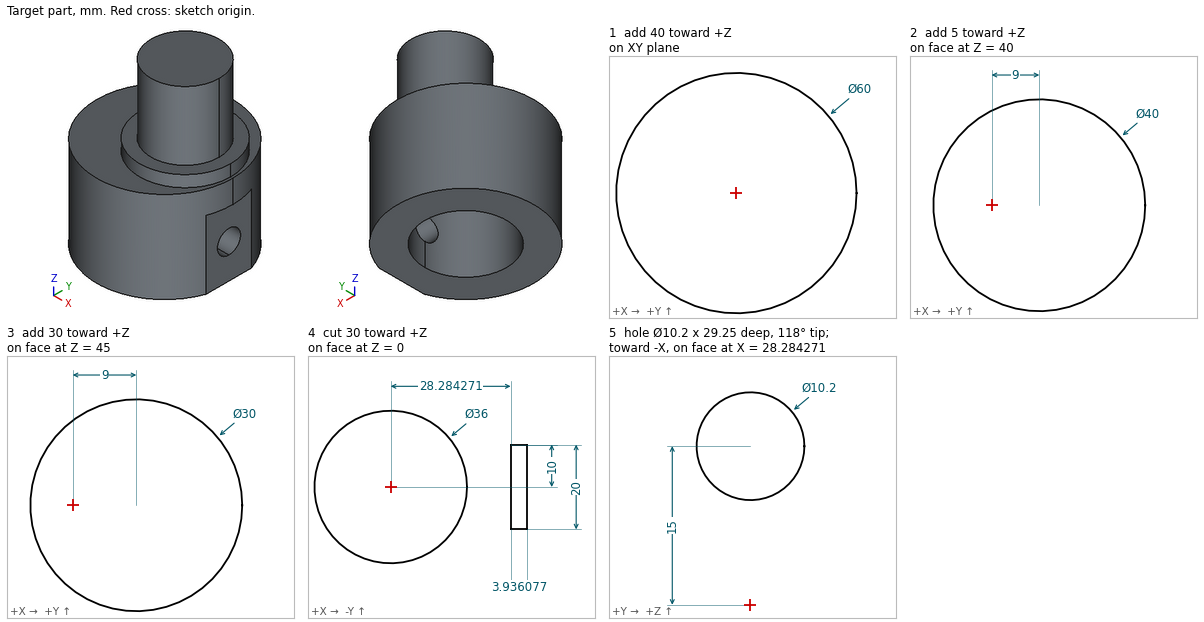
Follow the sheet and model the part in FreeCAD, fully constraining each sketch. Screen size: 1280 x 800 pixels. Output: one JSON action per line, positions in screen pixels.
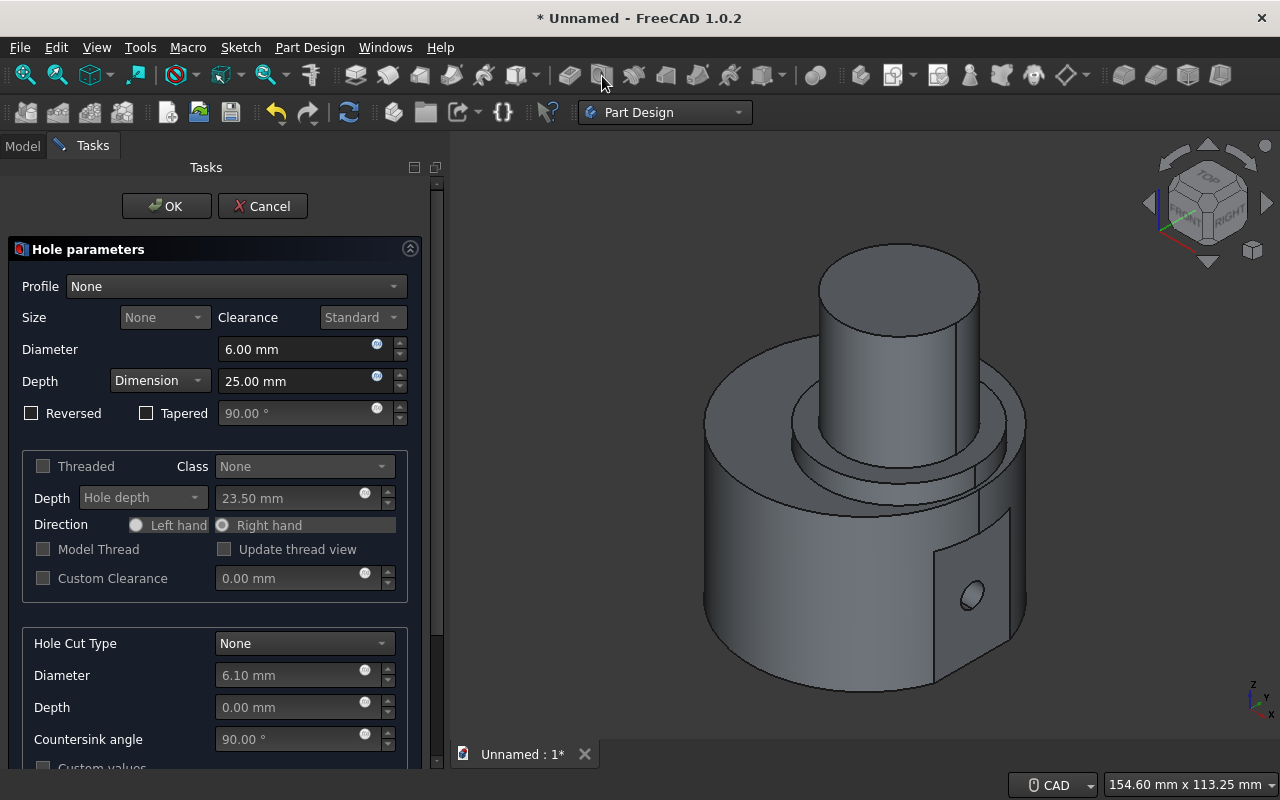
{"action": "triple_click", "coordinate": [305, 349]}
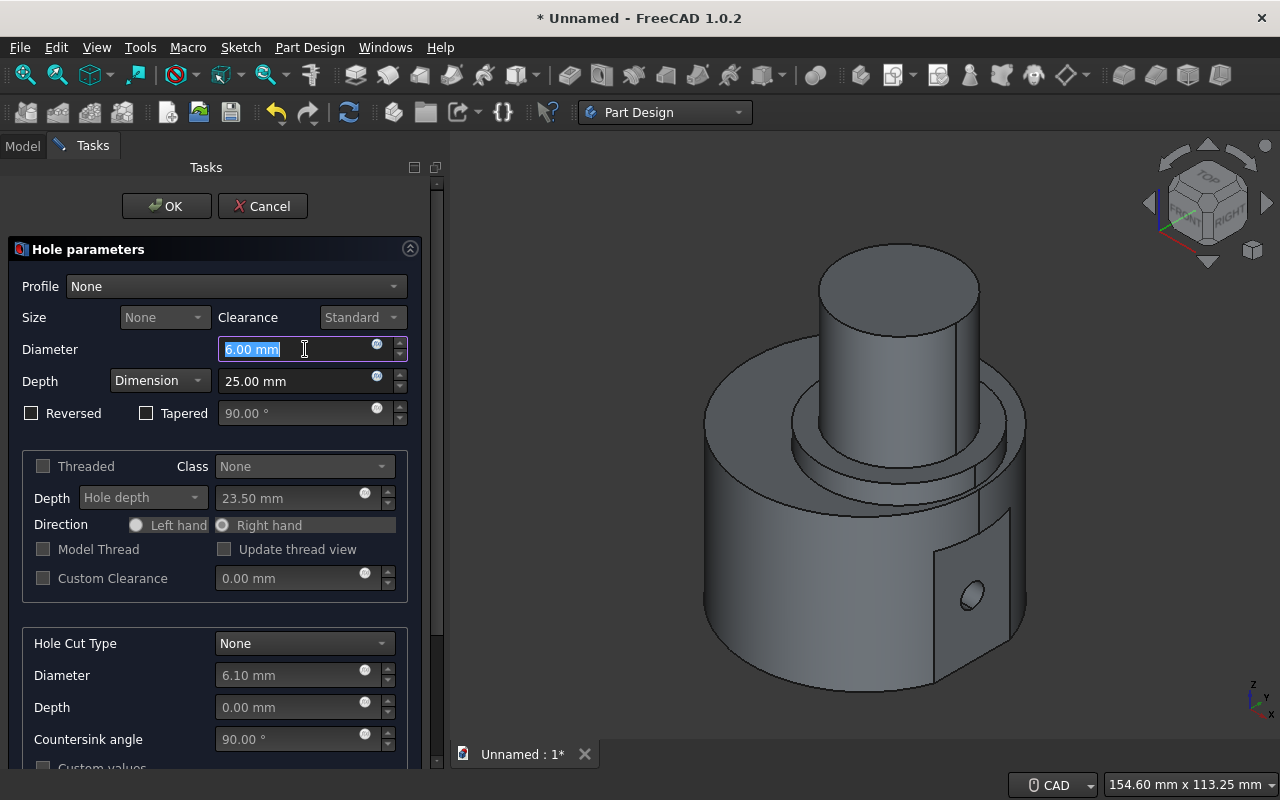
{"action": "type", "text": "10.2"}
{"action": "key", "text": "Tab"}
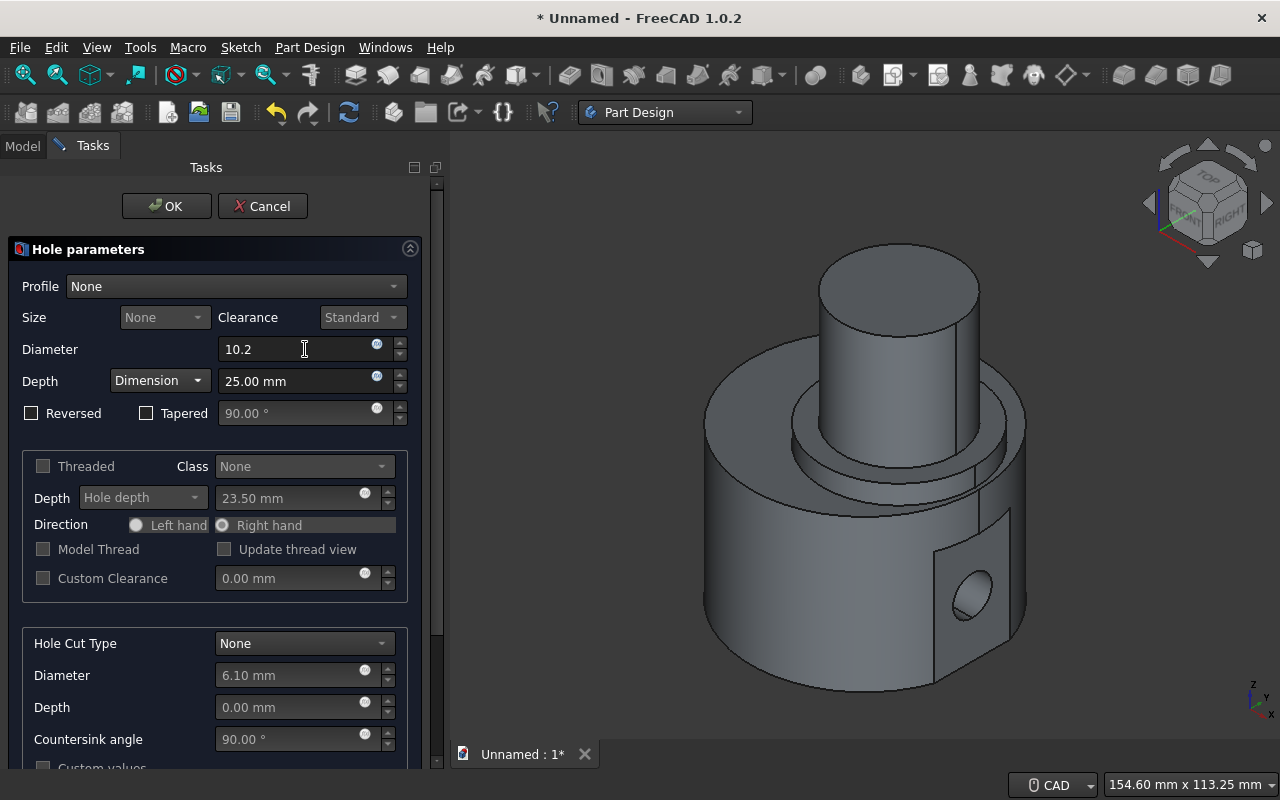
{"action": "triple_click", "coordinate": [305, 381]}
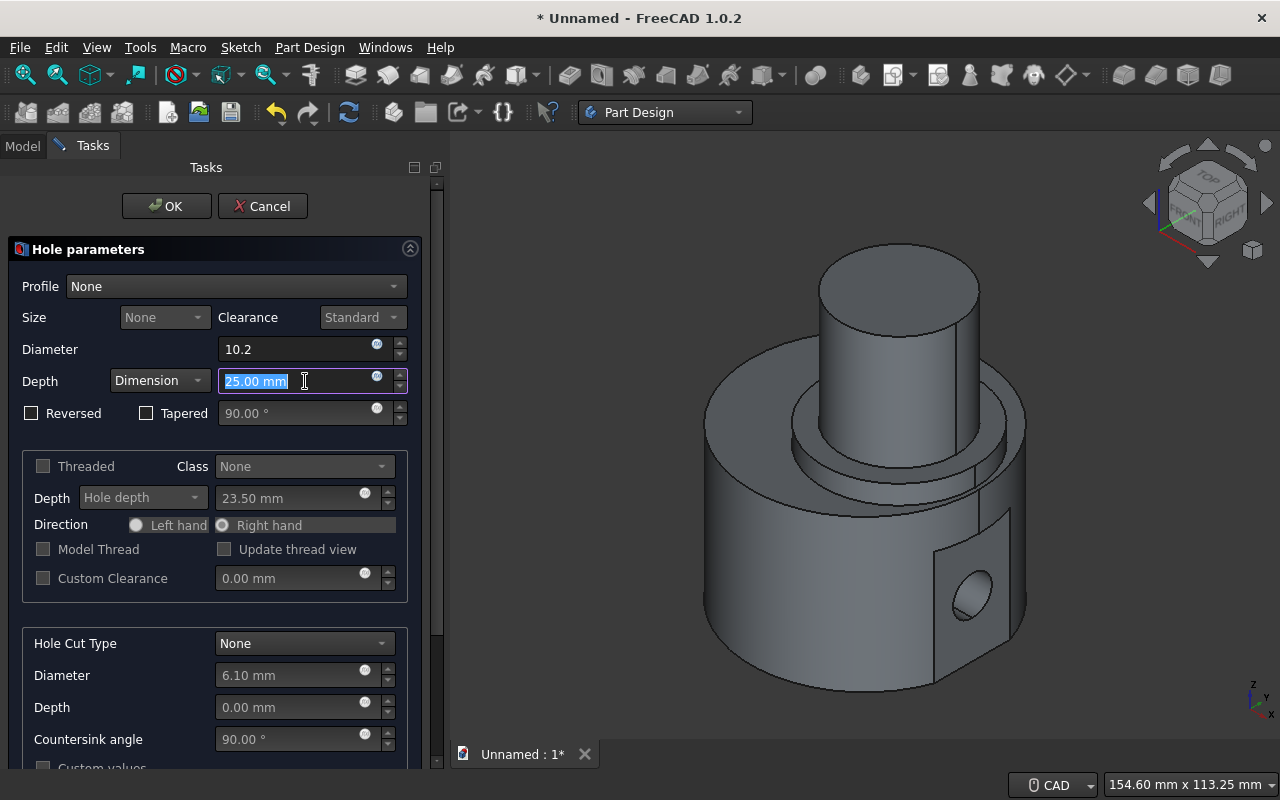
{"action": "type", "text": "29.25"}
{"action": "key", "text": "Tab"}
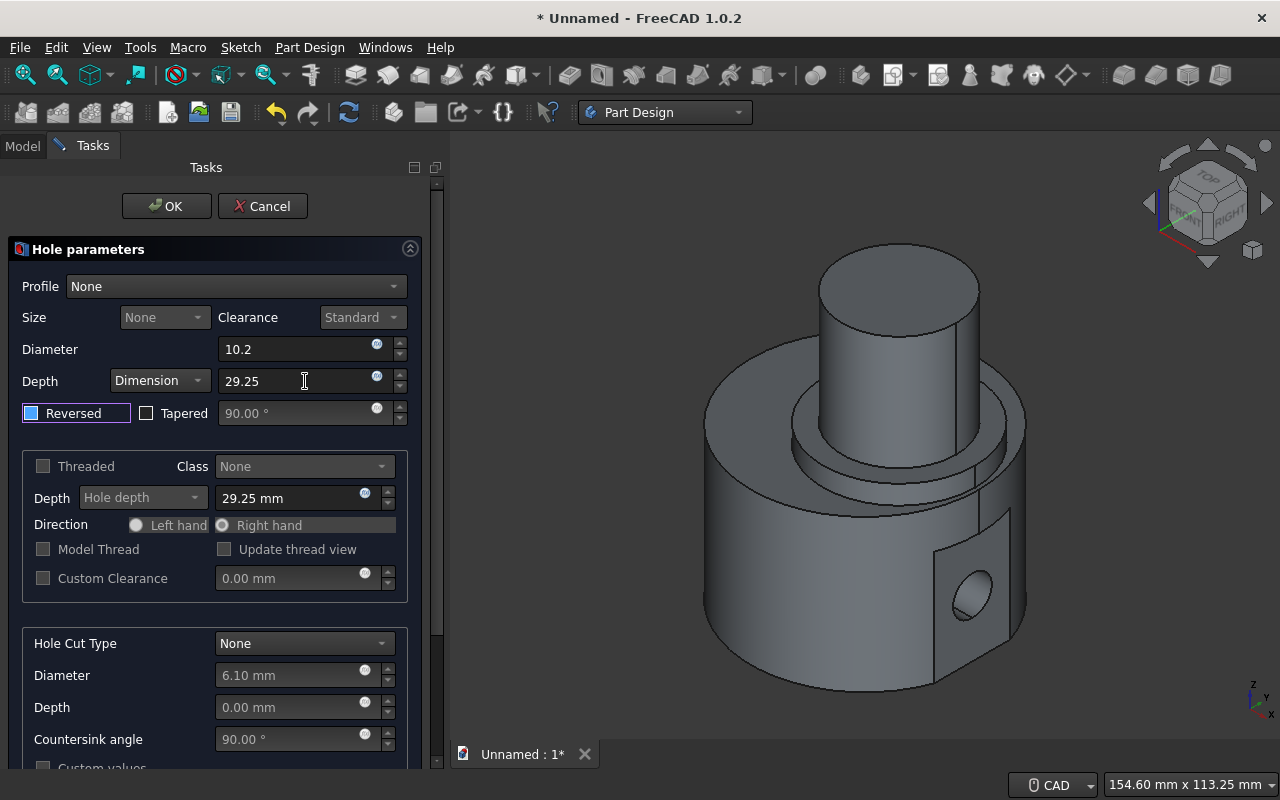
{"action": "left_click", "coordinate": [167, 206]}